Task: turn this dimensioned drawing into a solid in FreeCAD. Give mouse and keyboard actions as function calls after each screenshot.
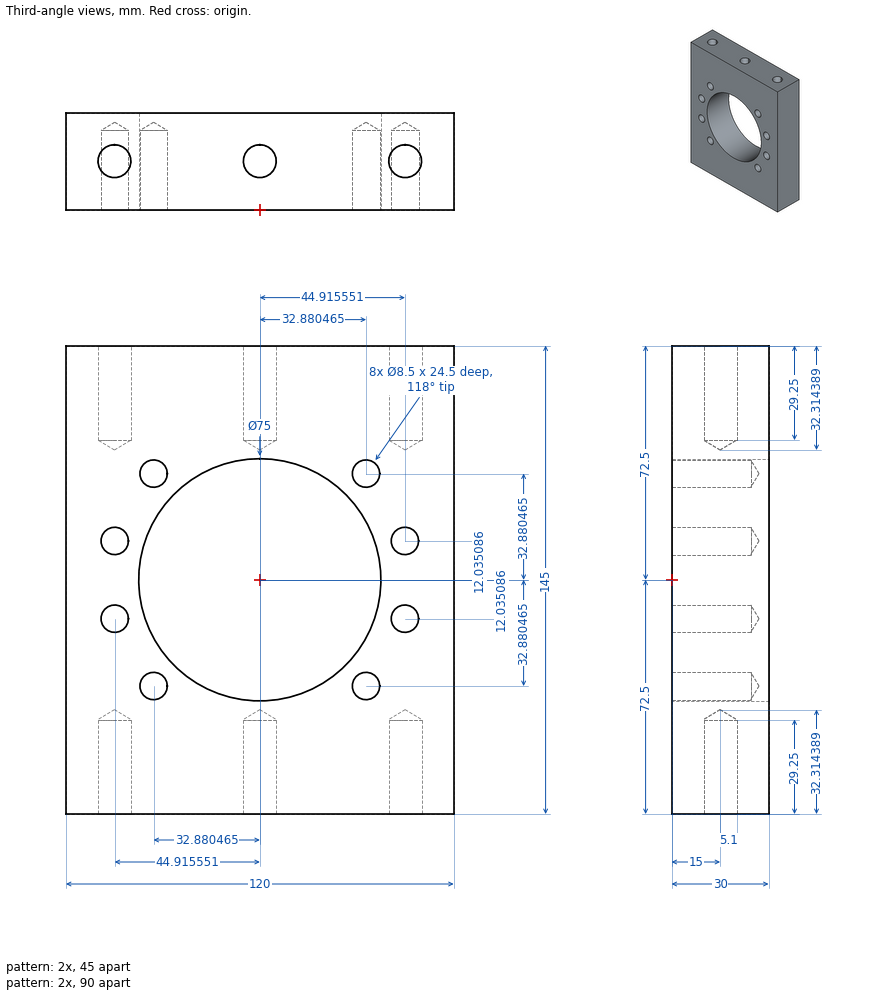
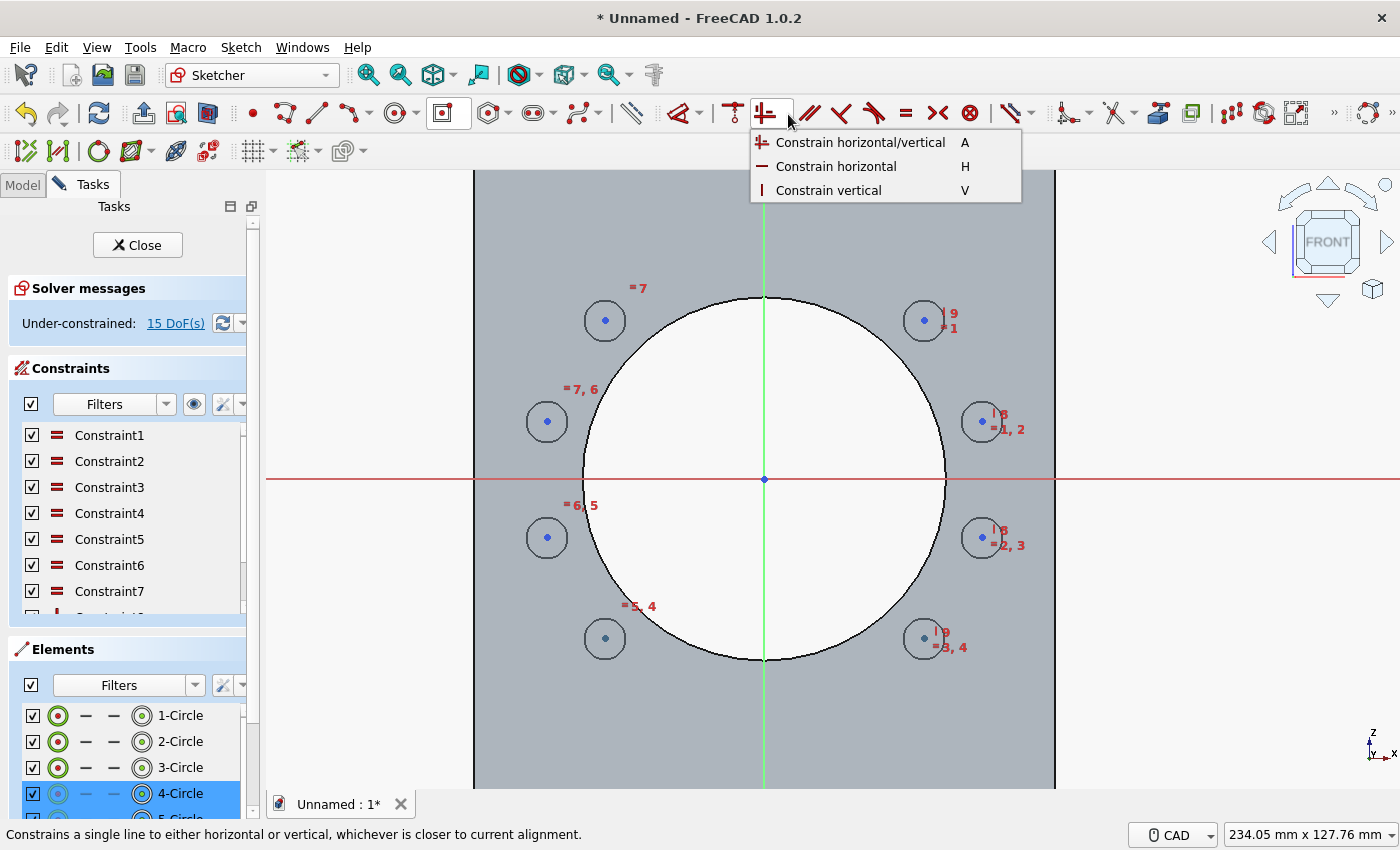
click(886, 166)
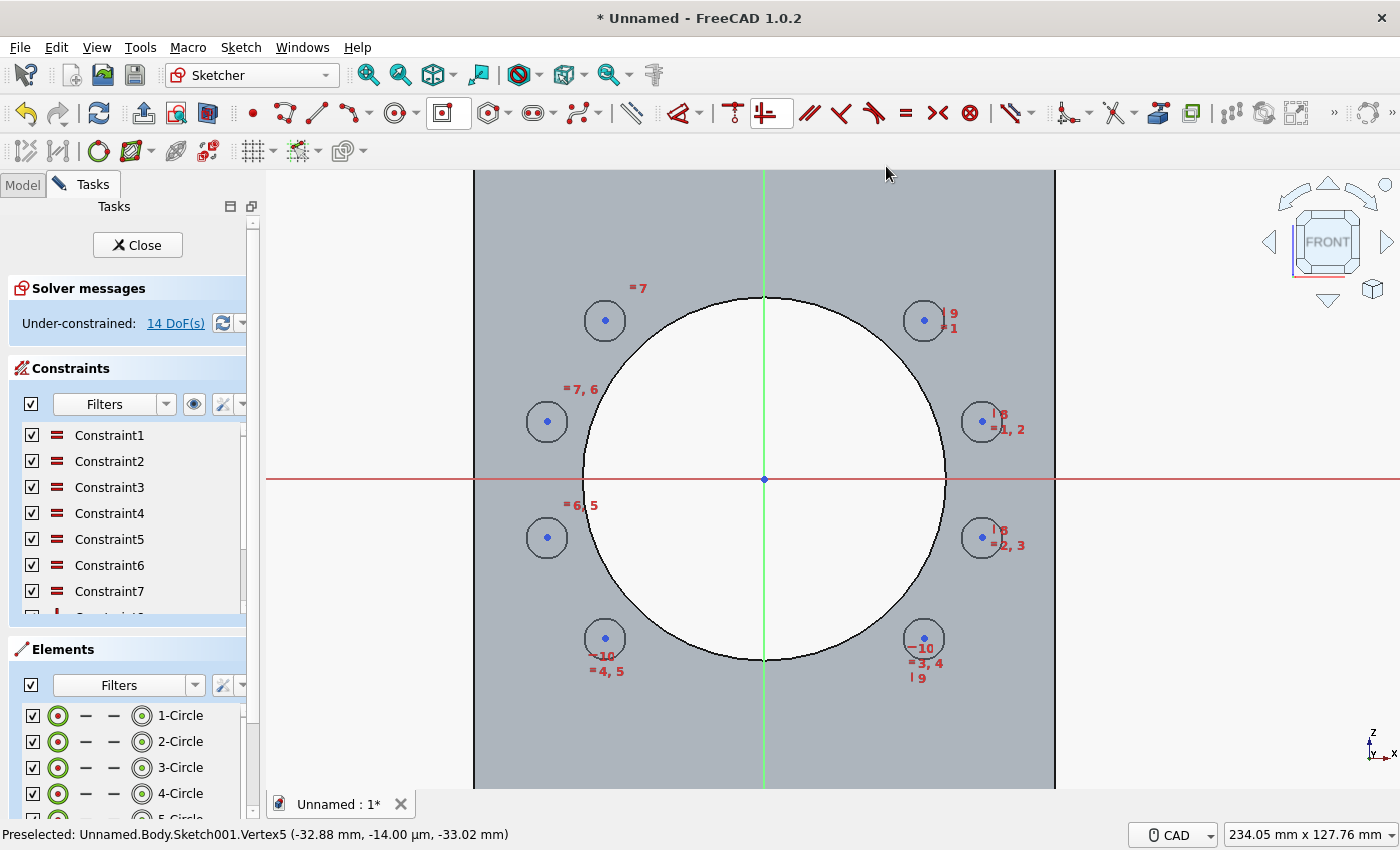
click(982, 538)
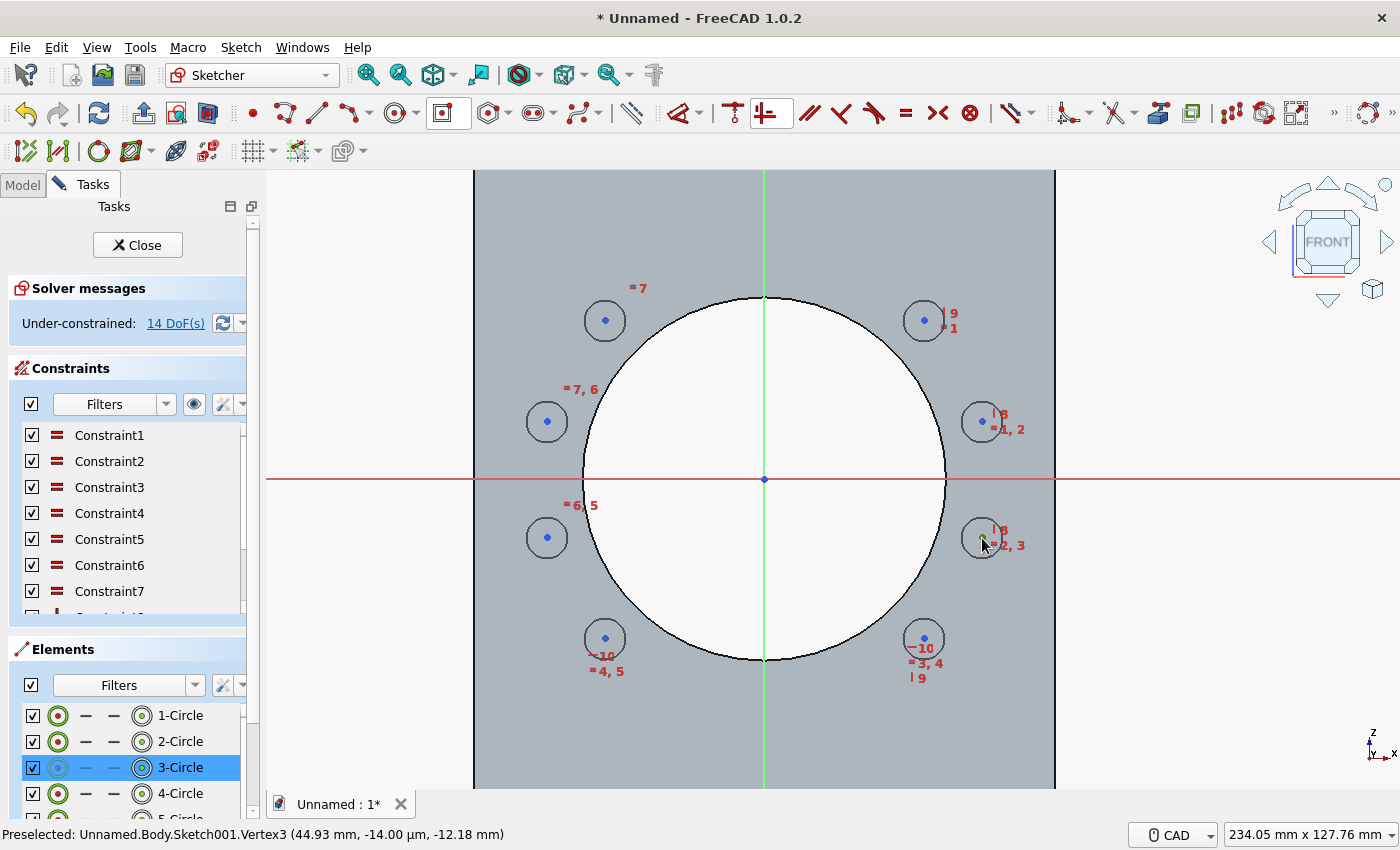
click(547, 538)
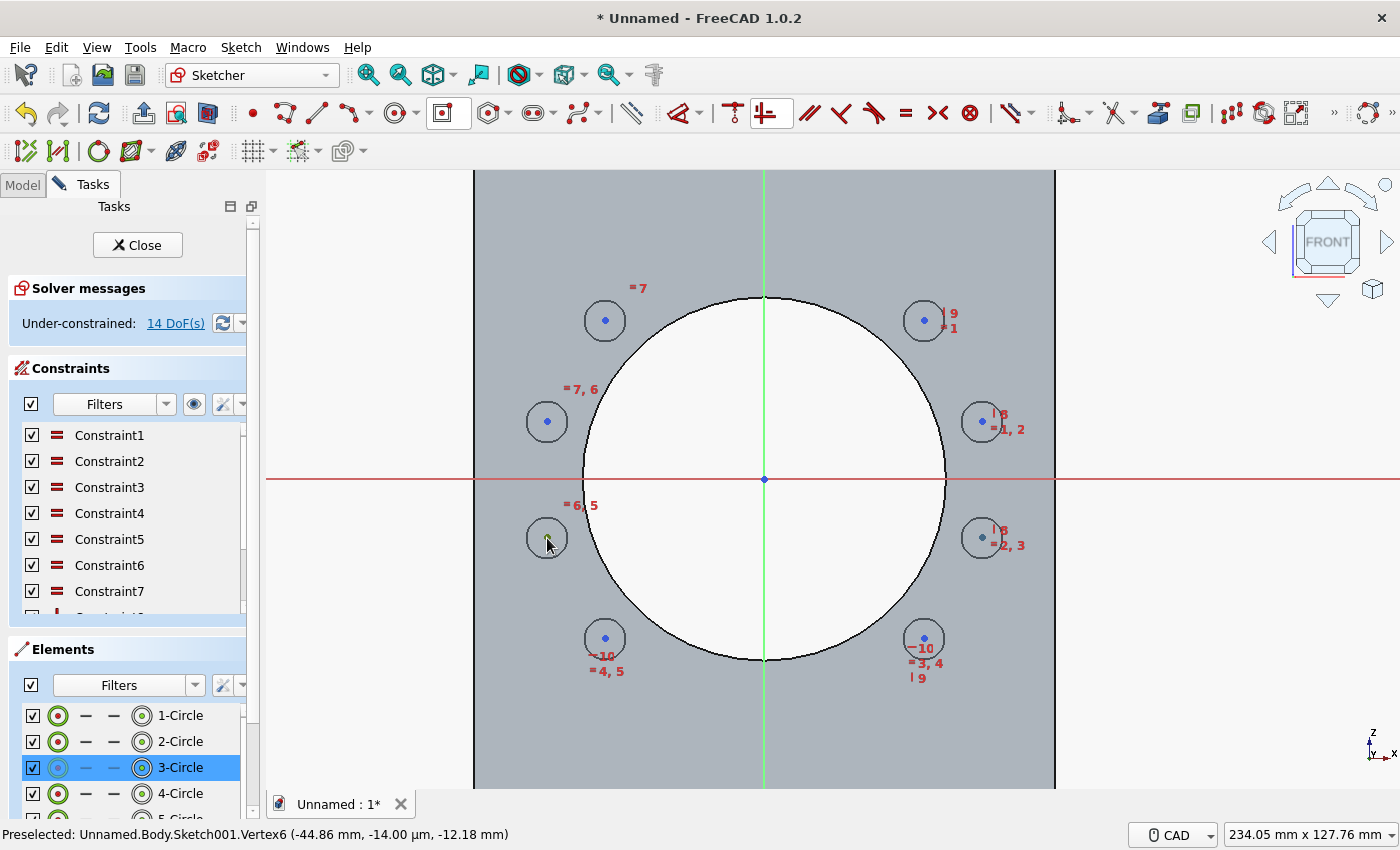
click(788, 114)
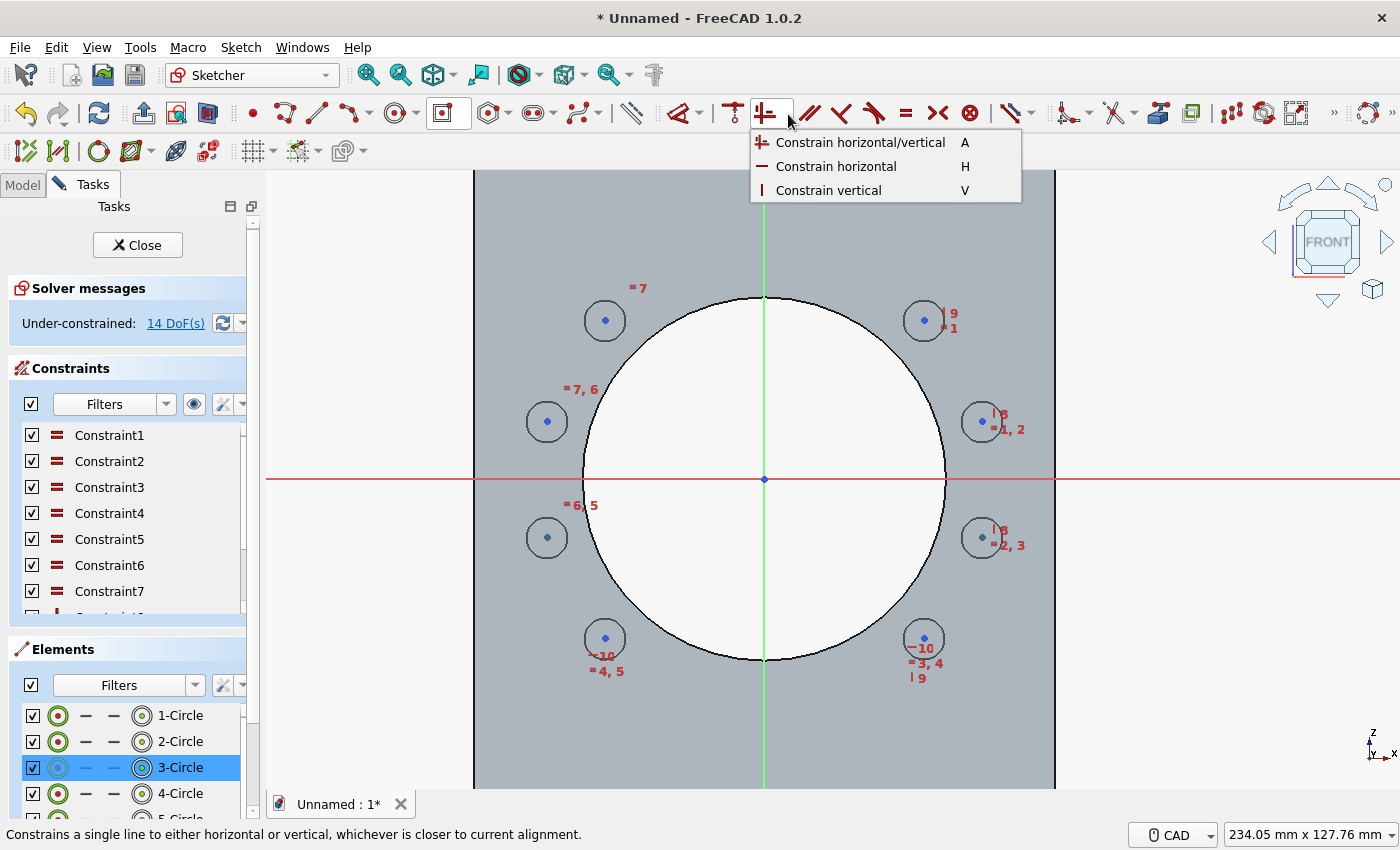
click(886, 166)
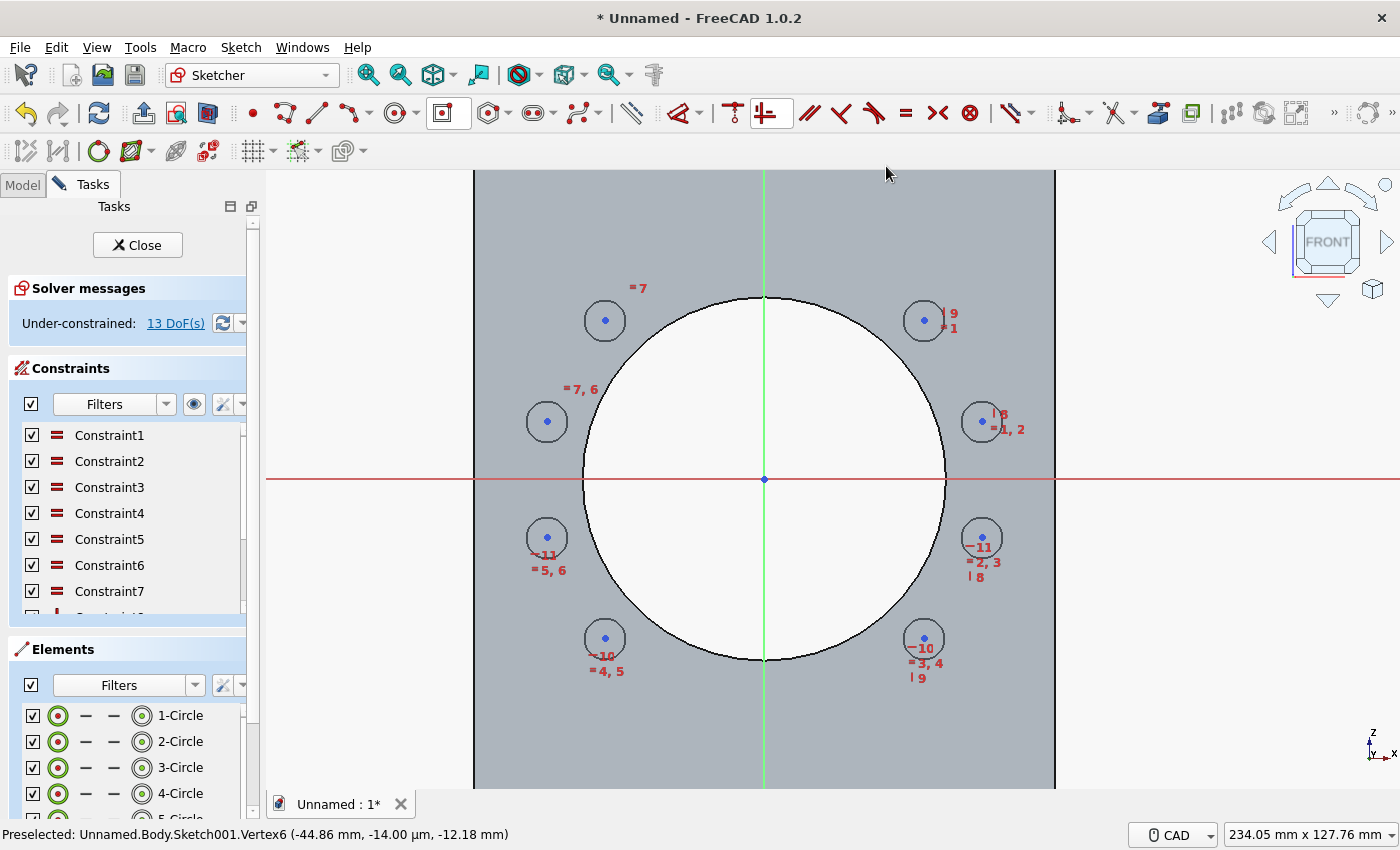
click(547, 538)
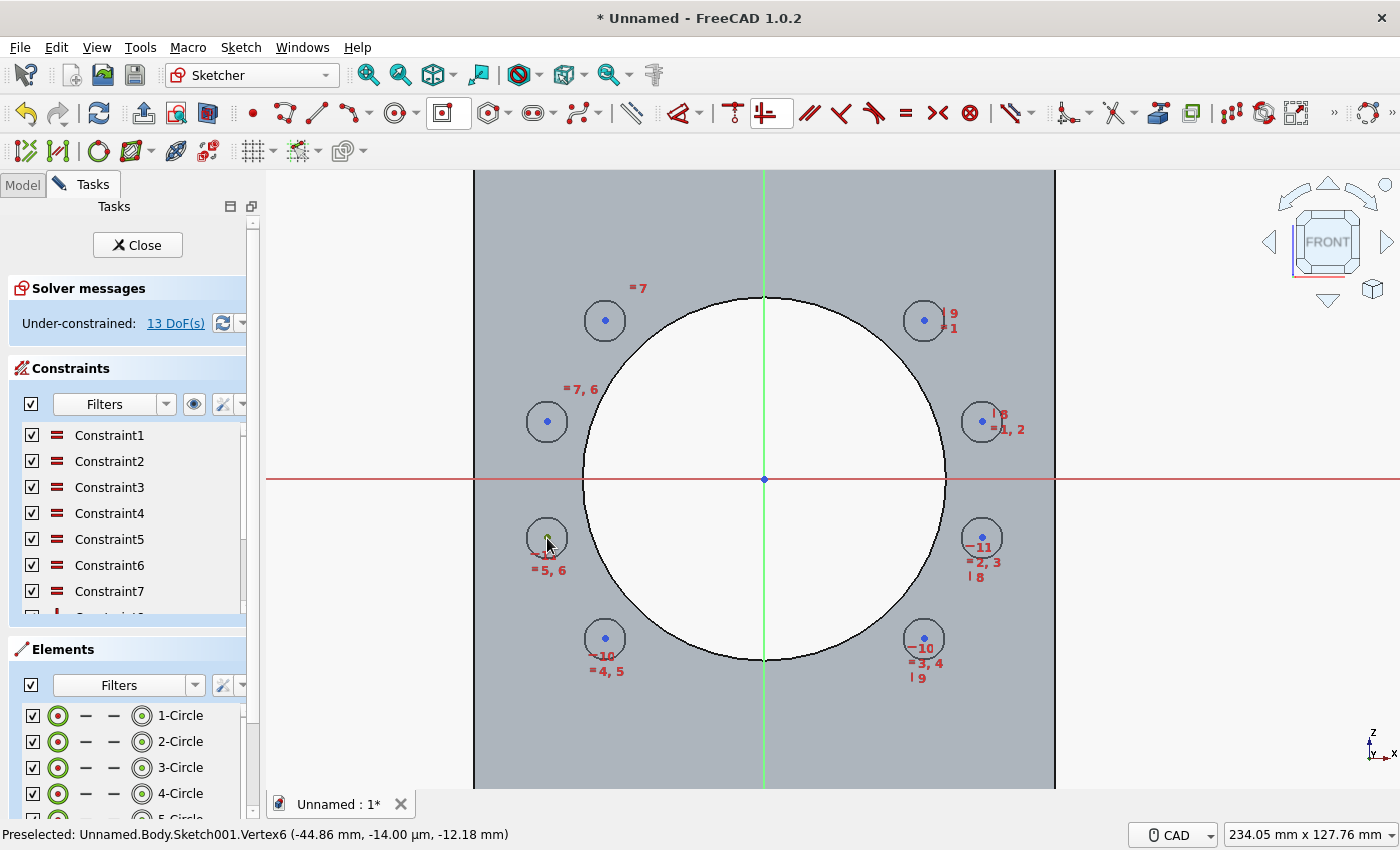
click(547, 422)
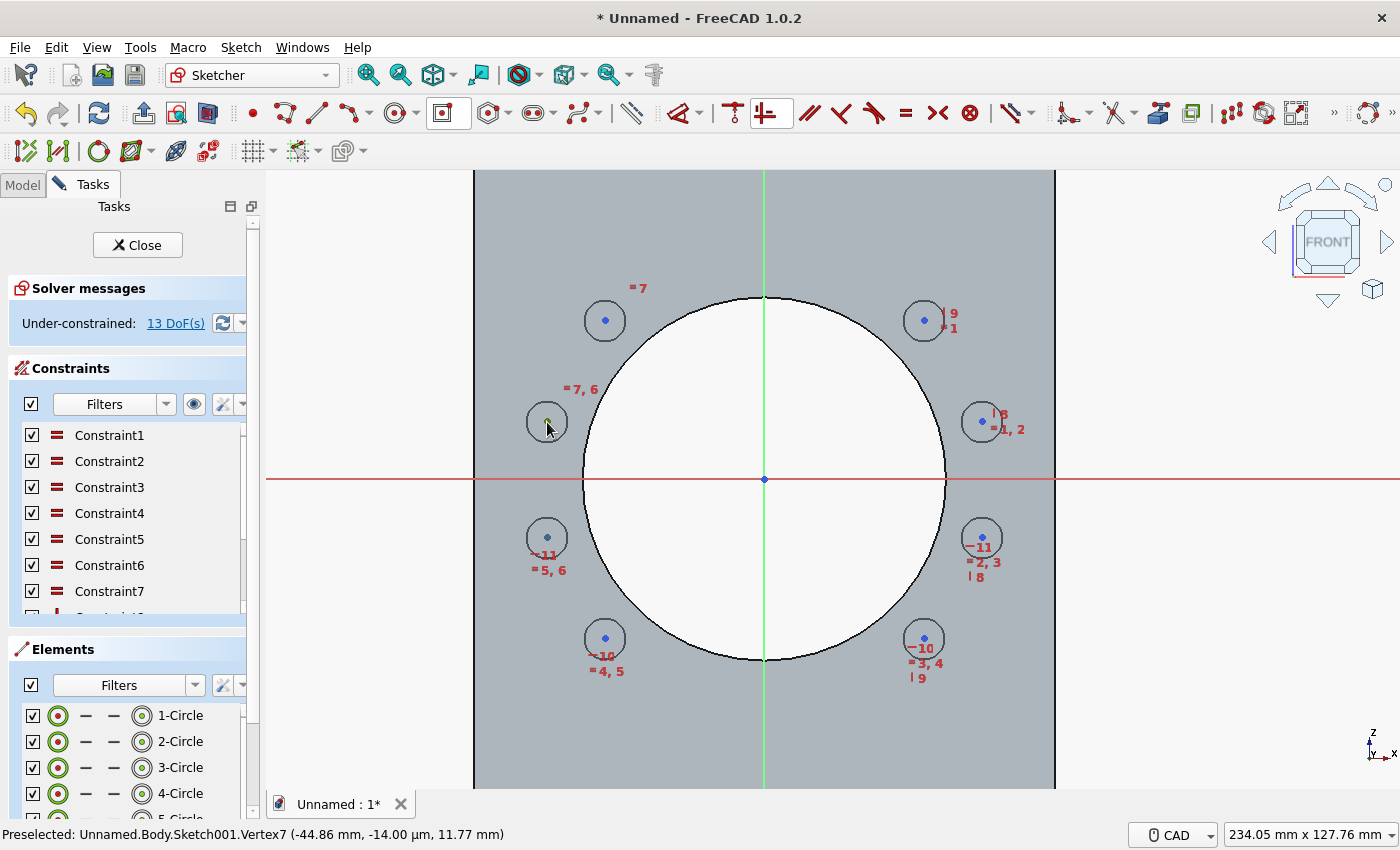
click(788, 114)